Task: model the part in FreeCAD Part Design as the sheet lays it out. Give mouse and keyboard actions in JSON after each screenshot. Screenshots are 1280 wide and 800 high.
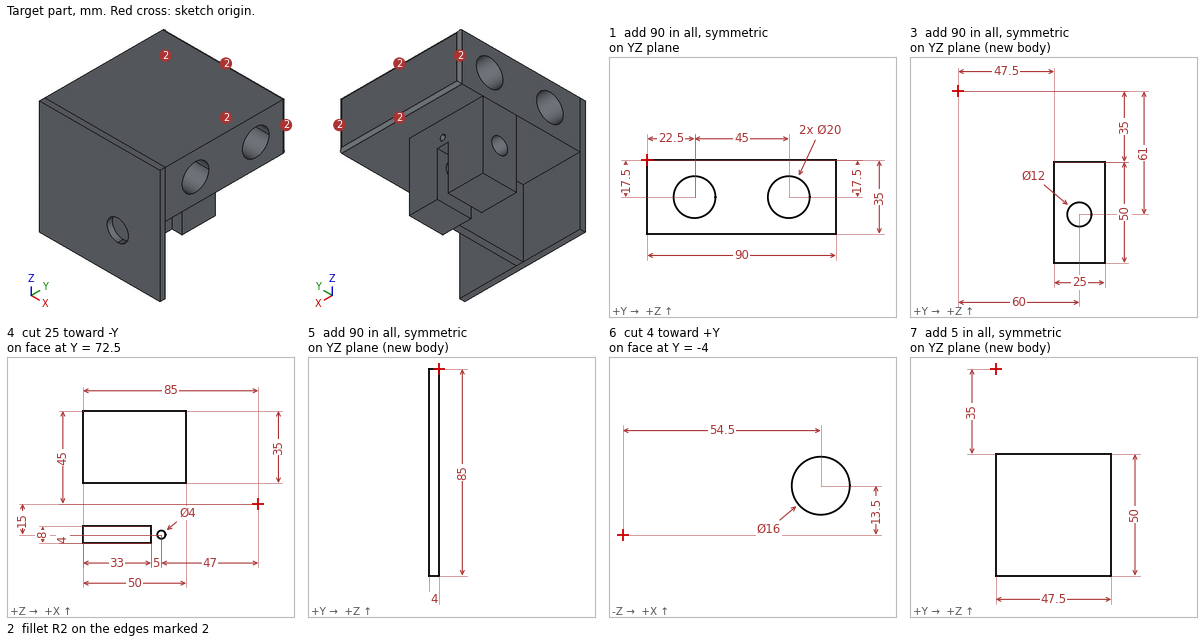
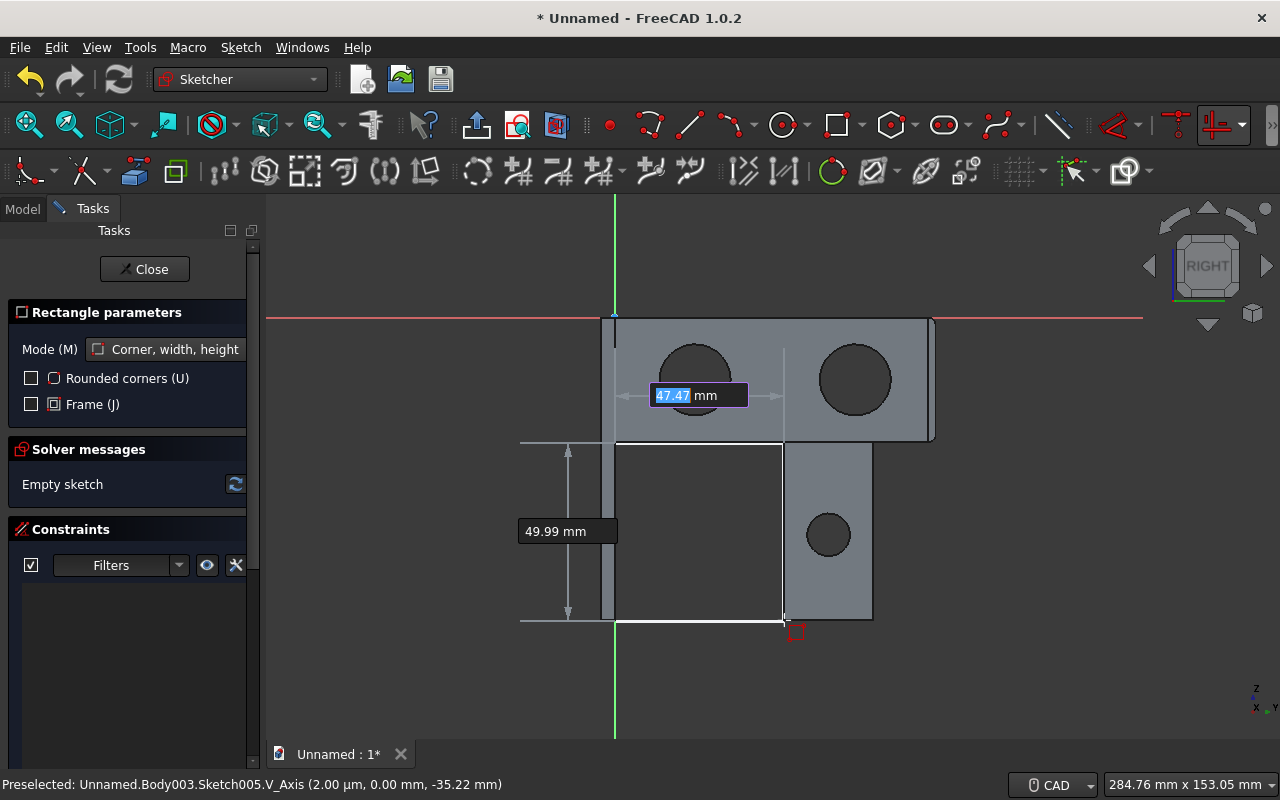
{"action": "type", "text": "47.5"}
{"action": "key", "text": "Tab"}
{"action": "type", "text": "50"}
{"action": "key", "text": "Return"}
{"action": "key", "text": "Escape"}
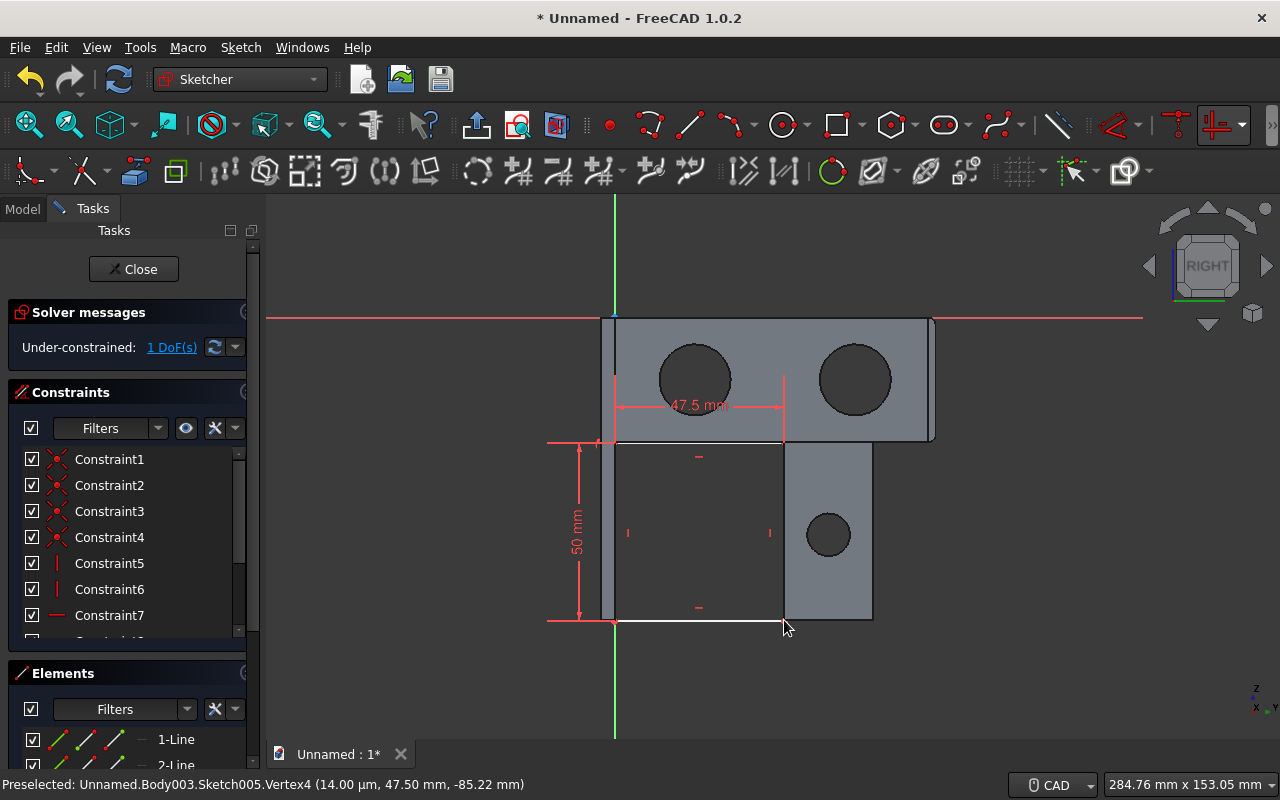
{"action": "left_click", "coordinate": [1114, 126]}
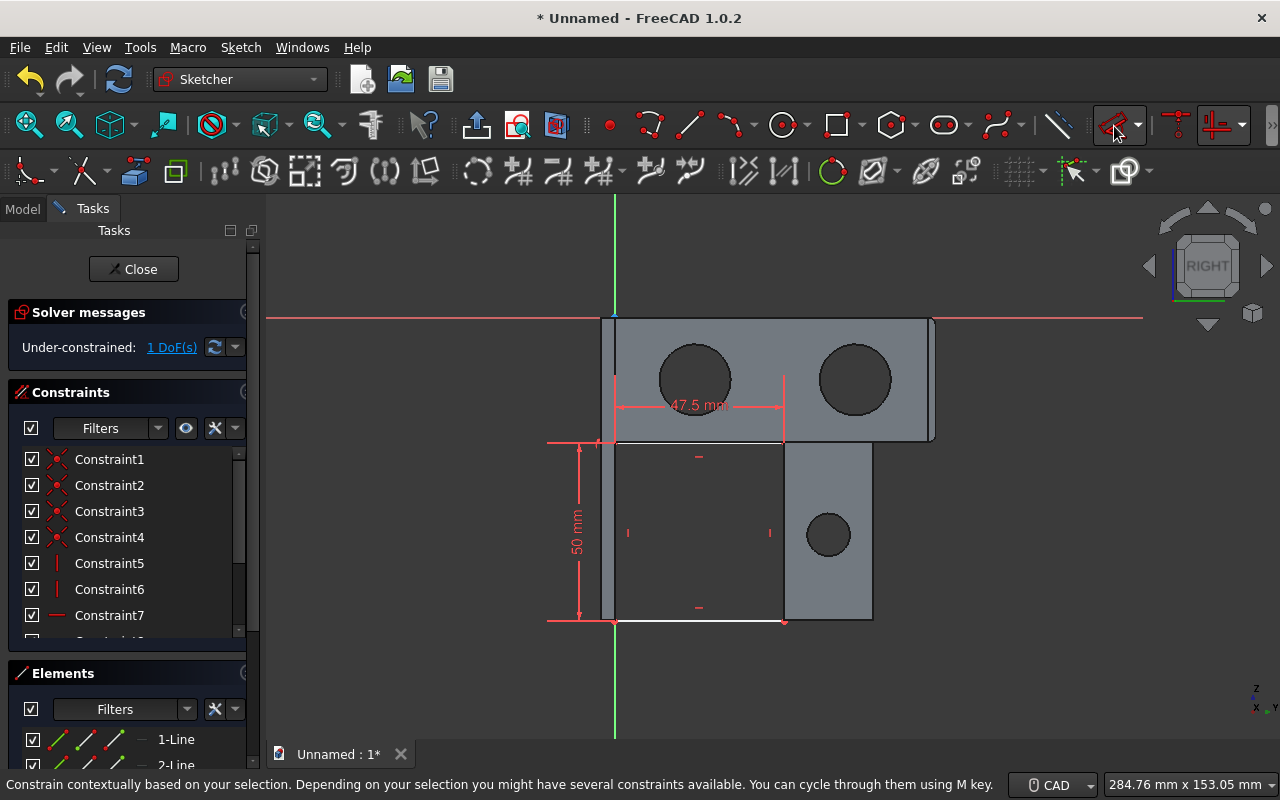
{"action": "left_click", "coordinate": [615, 443]}
{"action": "left_click", "coordinate": [581, 380]}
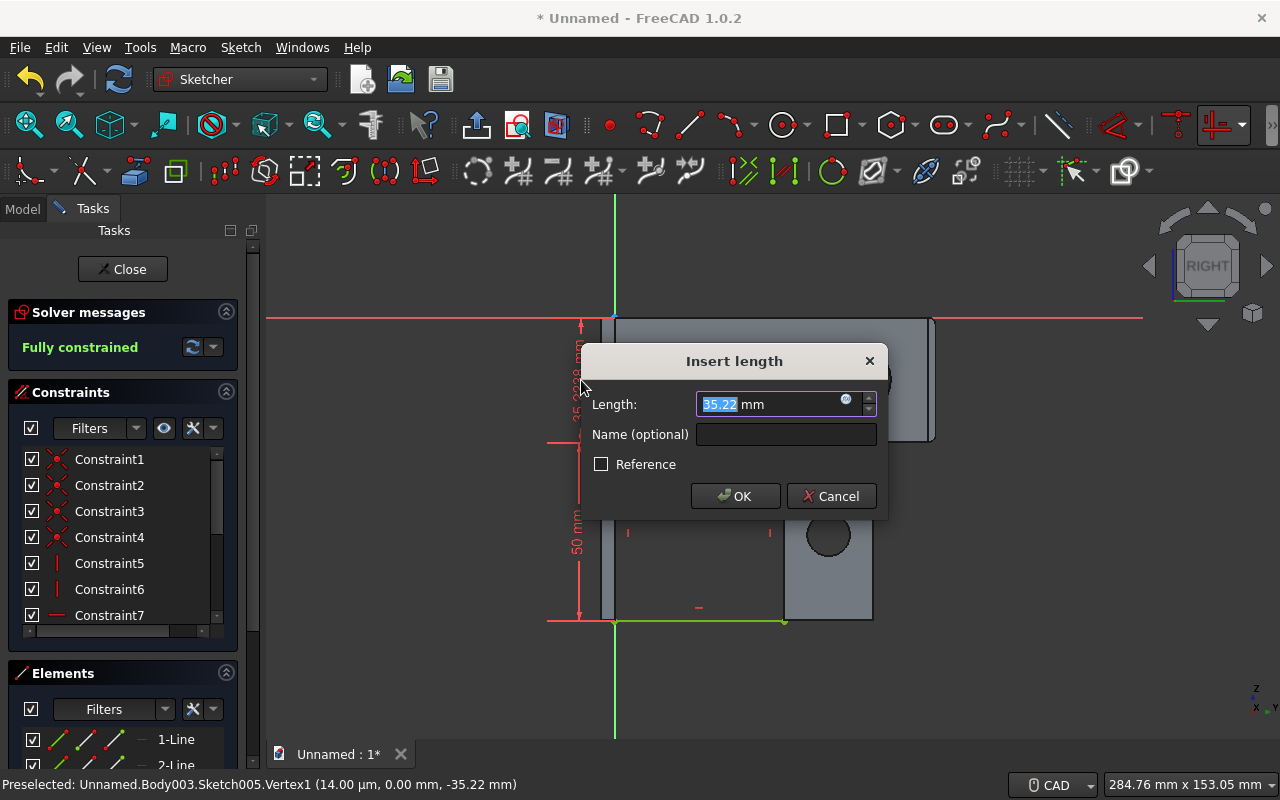
{"action": "type", "text": "35"}
{"action": "key", "text": "Return"}
{"action": "key", "text": "Escape"}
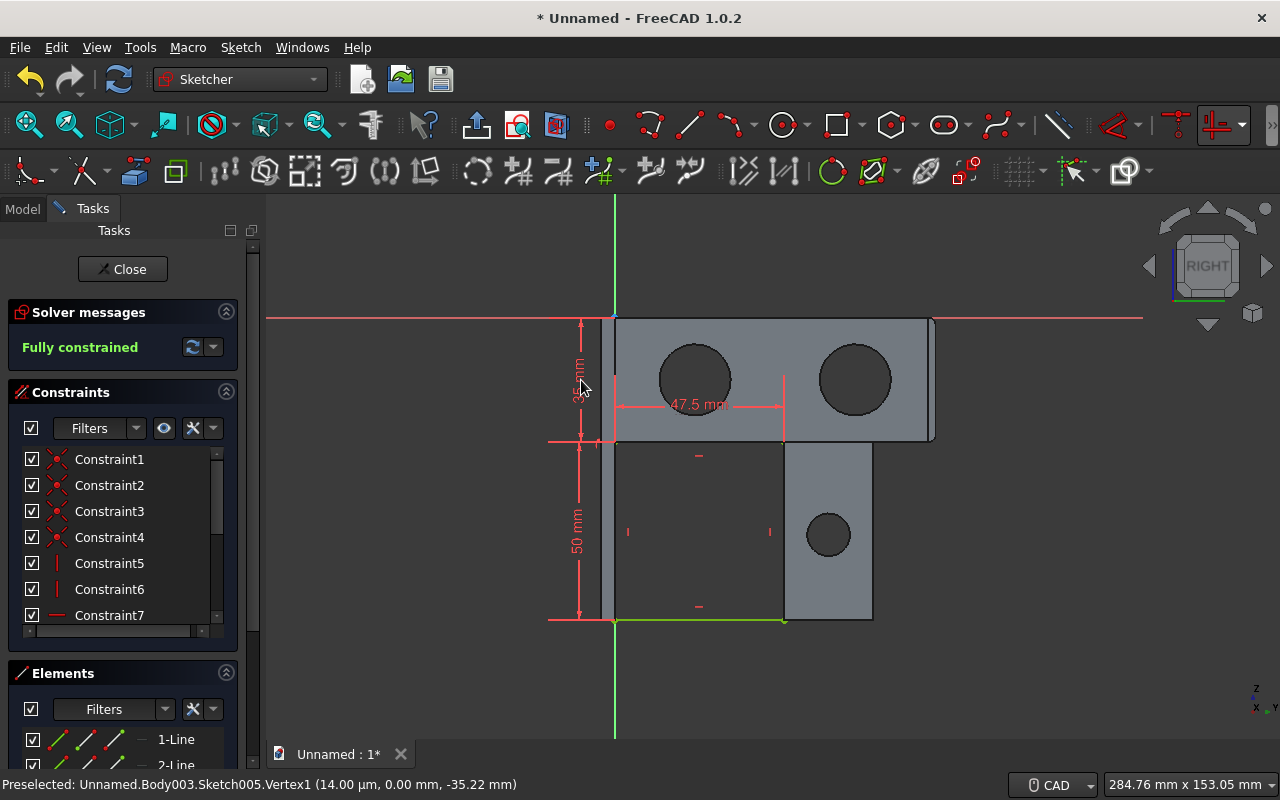
{"action": "left_click", "coordinate": [123, 269]}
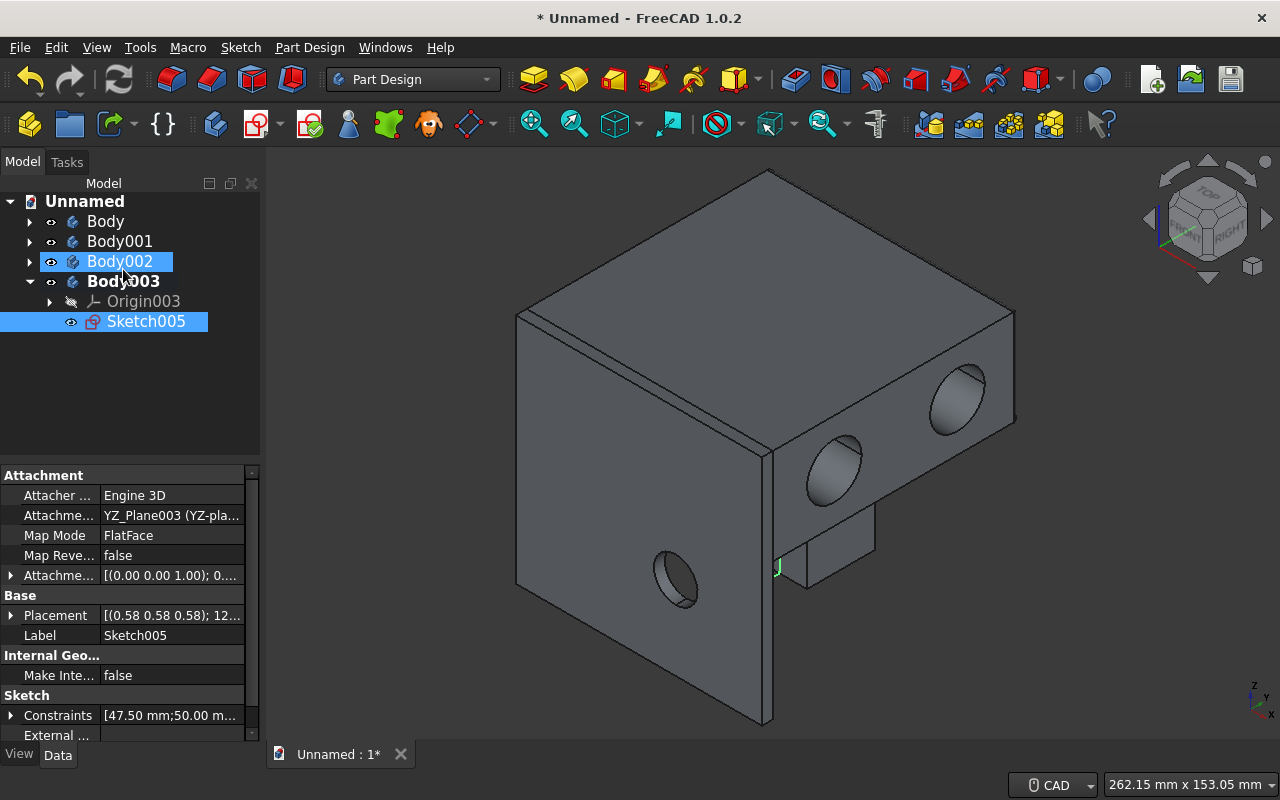
{"action": "left_click", "coordinate": [534, 80]}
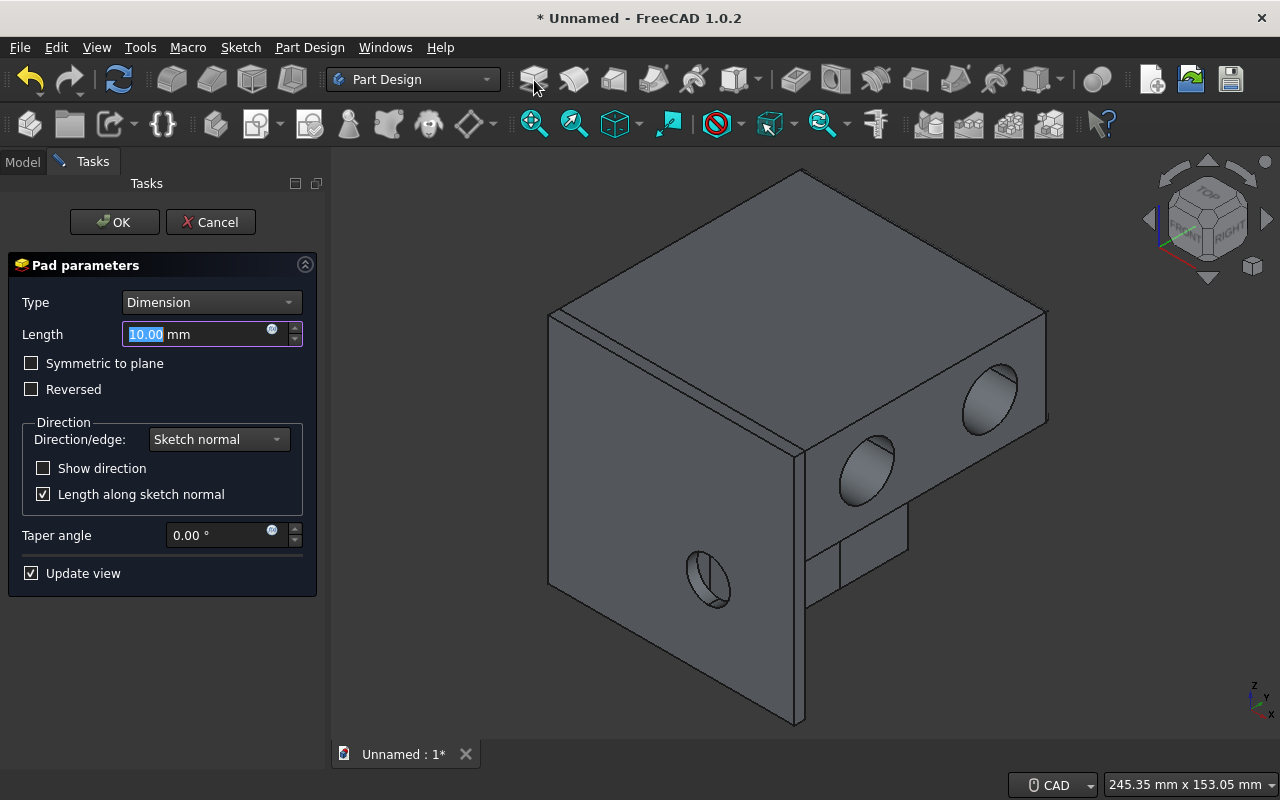
{"action": "type", "text": "5"}
{"action": "key", "text": "Tab"}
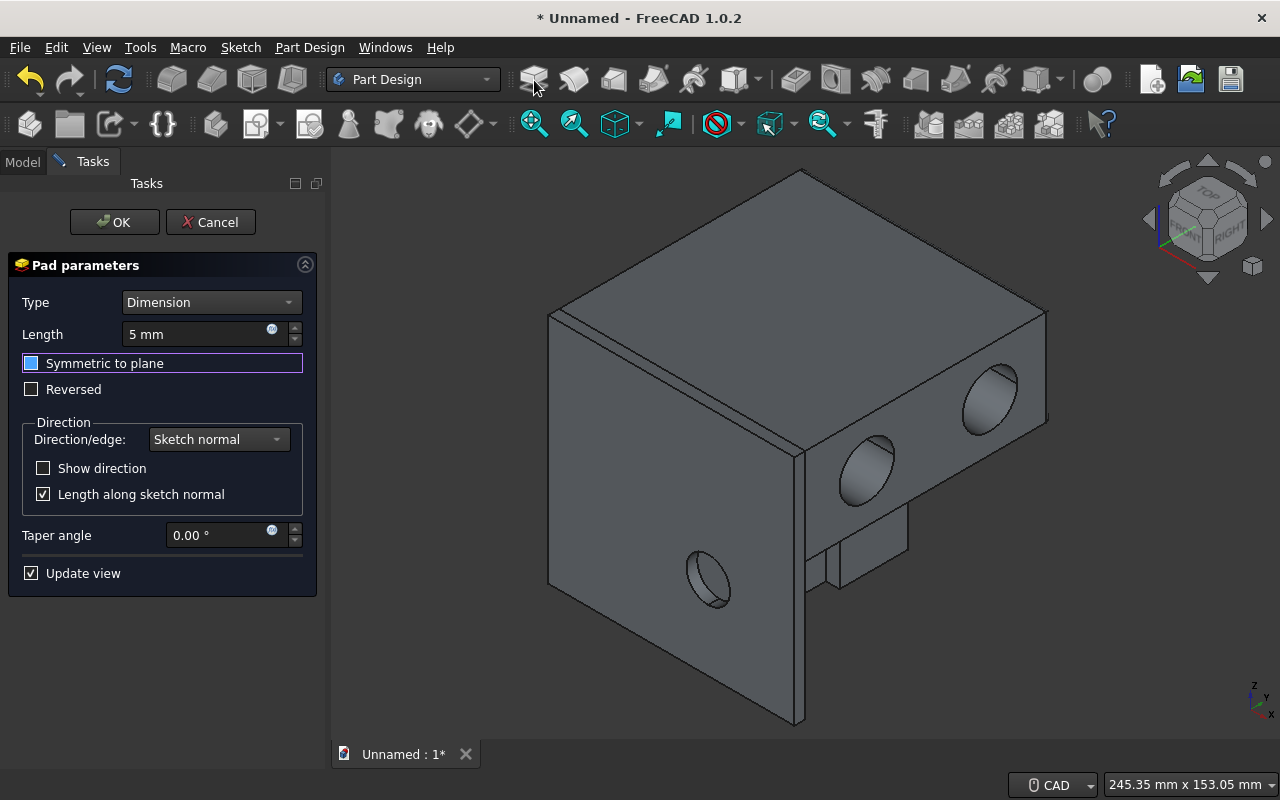
{"action": "left_click", "coordinate": [30, 363]}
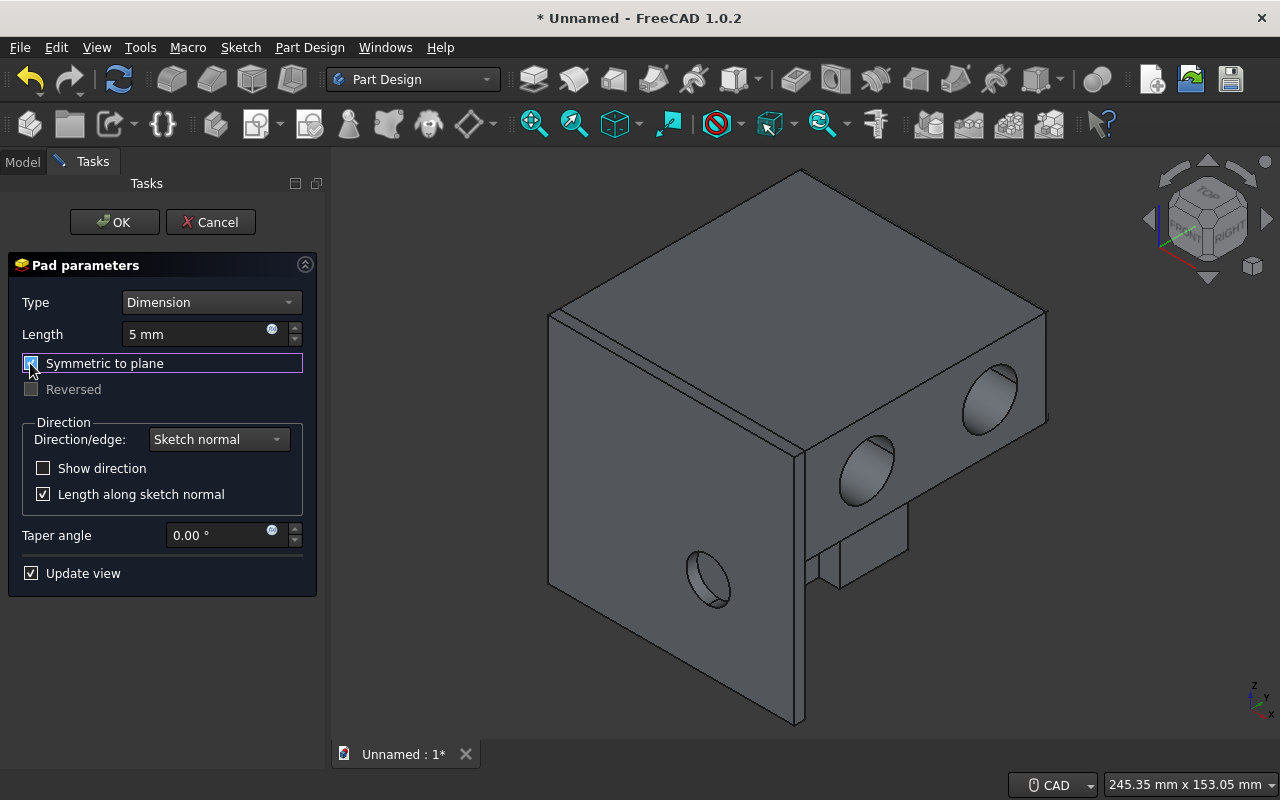
{"action": "left_click", "coordinate": [115, 222]}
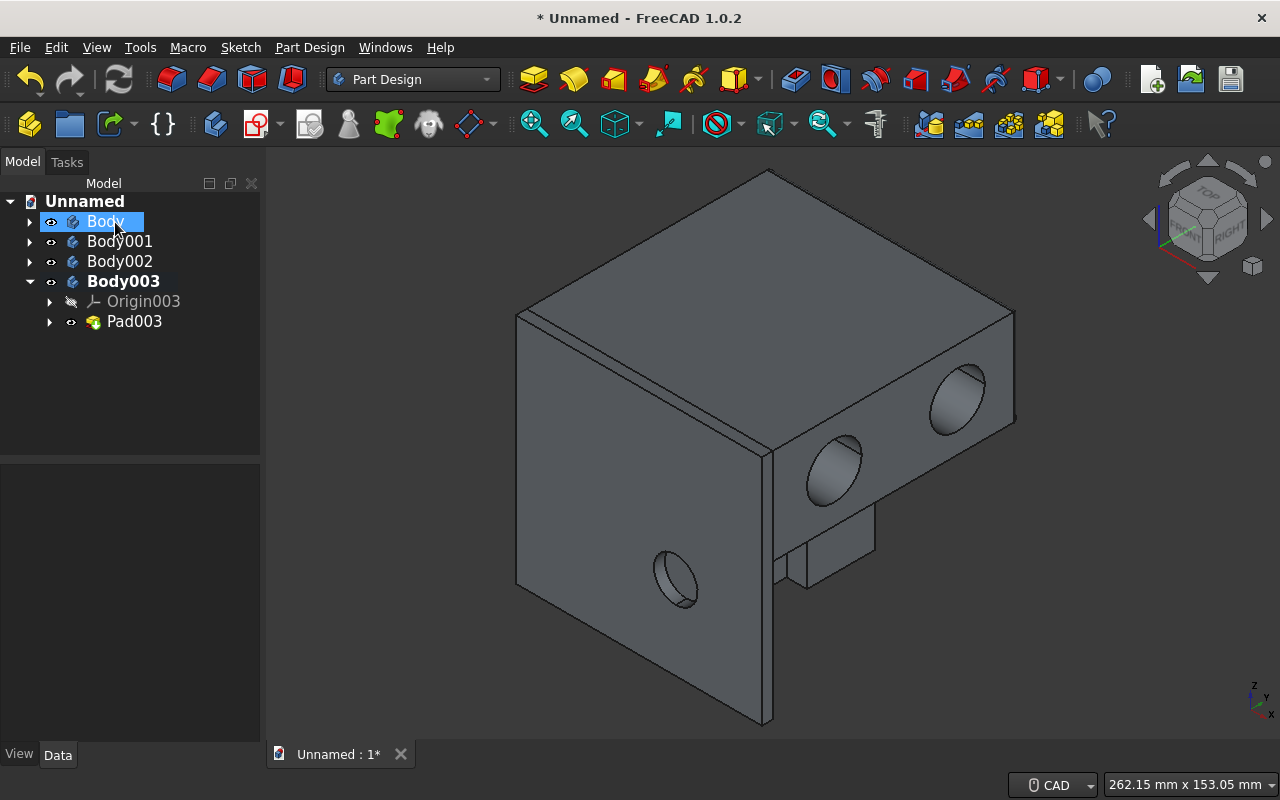
{"action": "left_click", "coordinate": [536, 124]}